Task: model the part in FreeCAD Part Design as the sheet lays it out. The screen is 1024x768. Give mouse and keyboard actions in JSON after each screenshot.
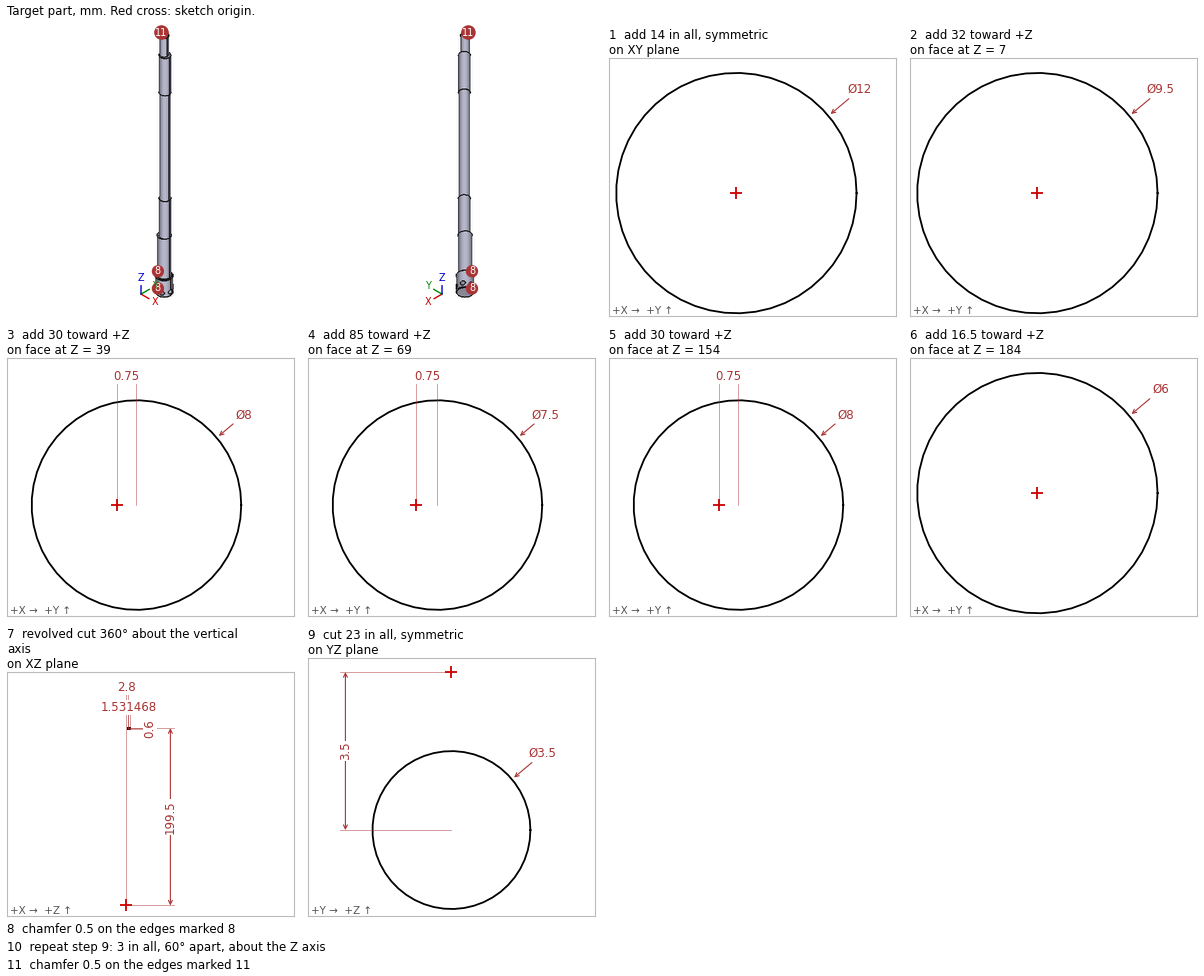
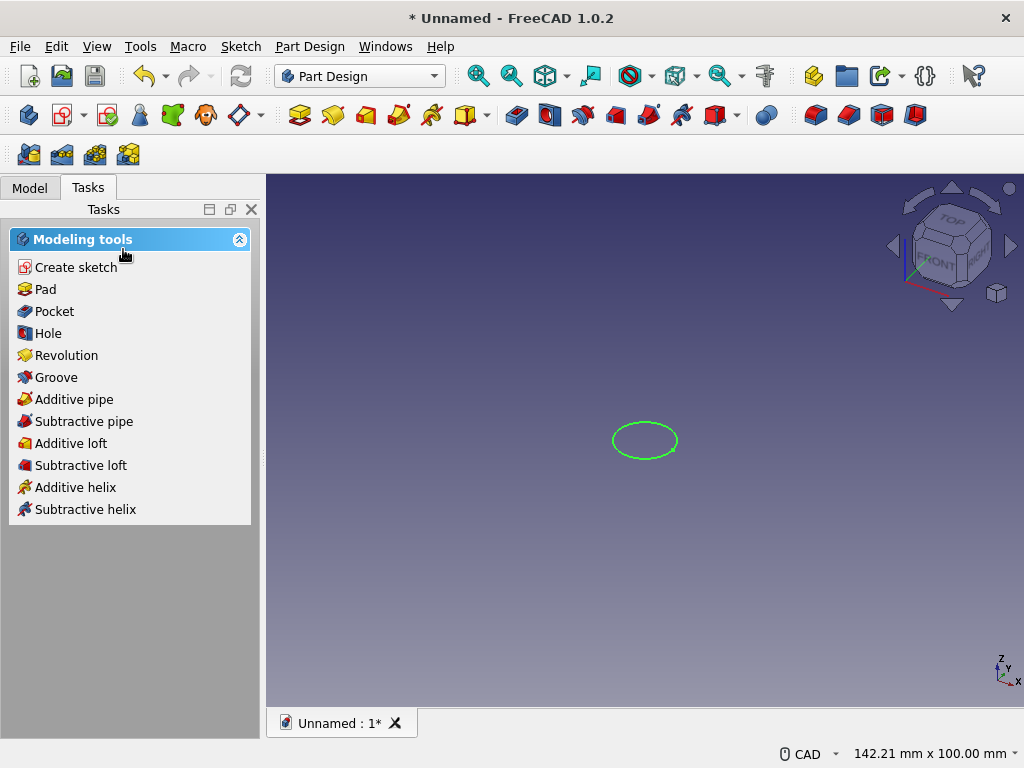
{"action": "left_click", "coordinate": [300, 116]}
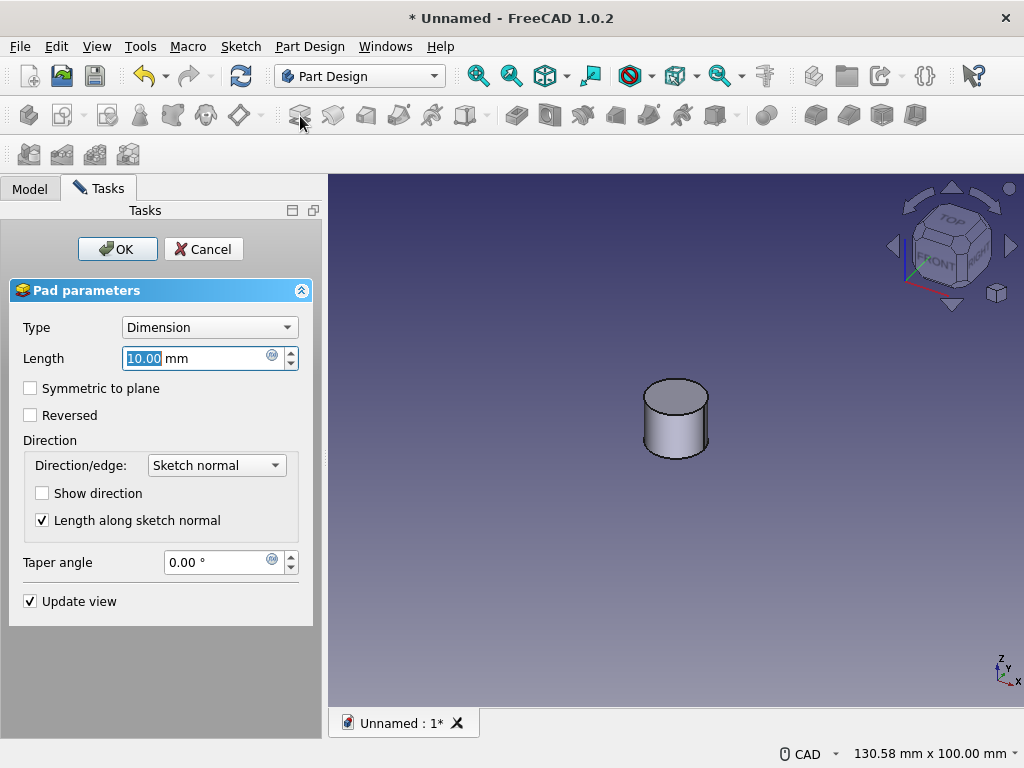
{"action": "type", "text": "14"}
{"action": "key", "text": "Tab"}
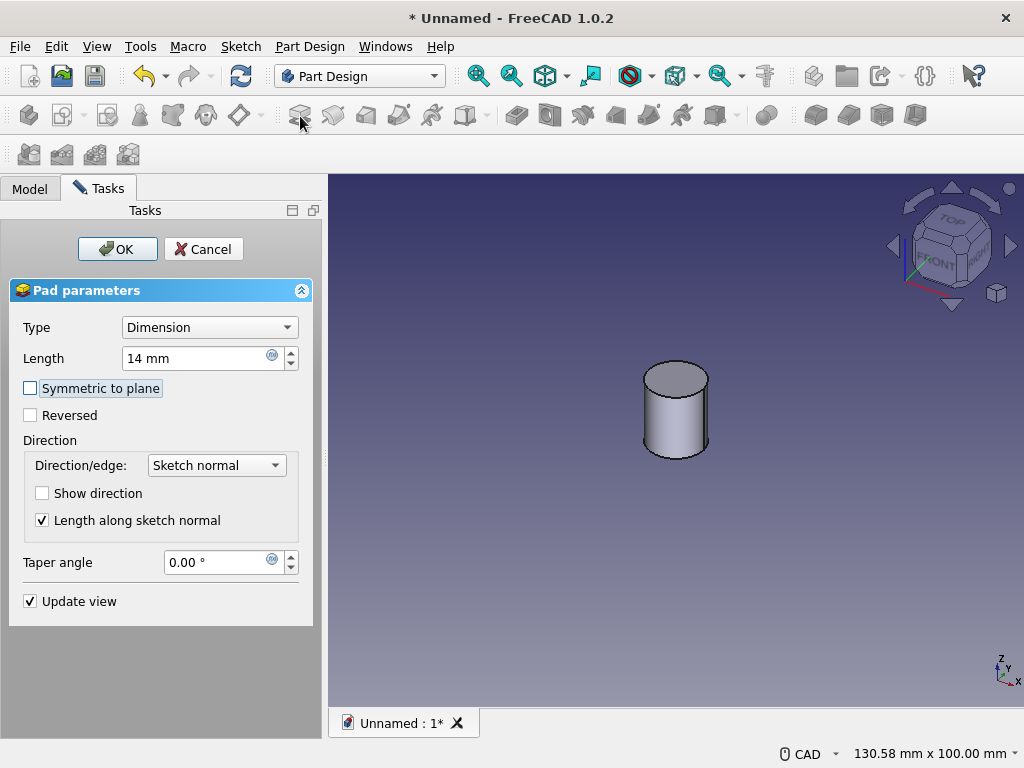
{"action": "left_click", "coordinate": [31, 388]}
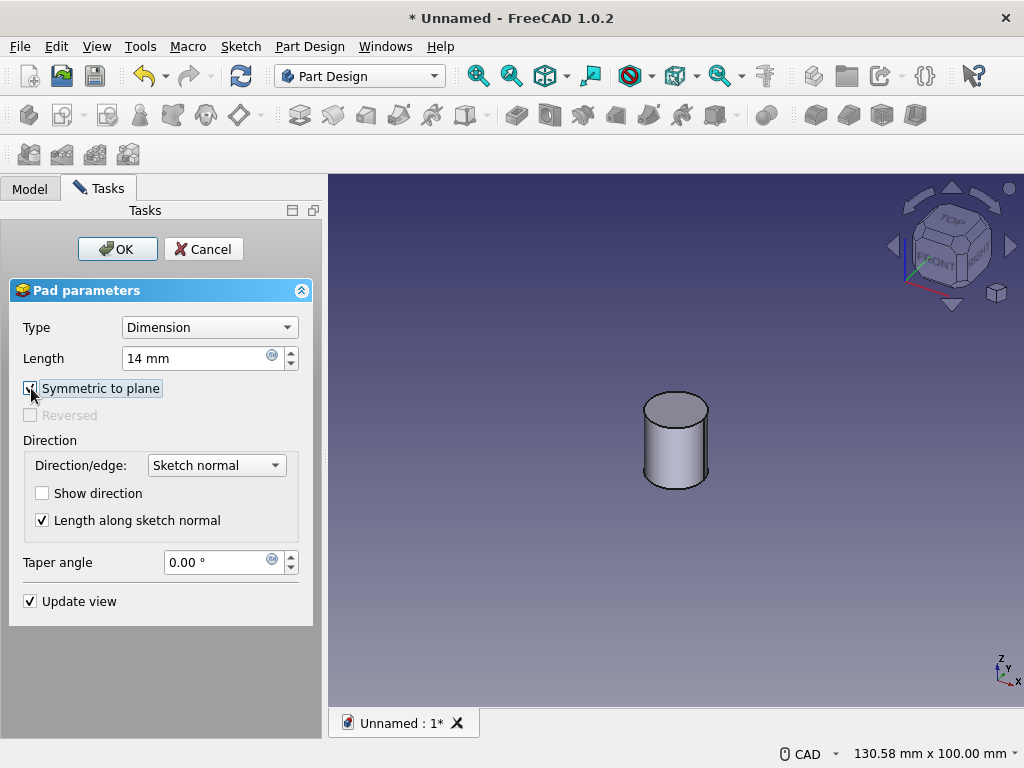
{"action": "left_click", "coordinate": [118, 249]}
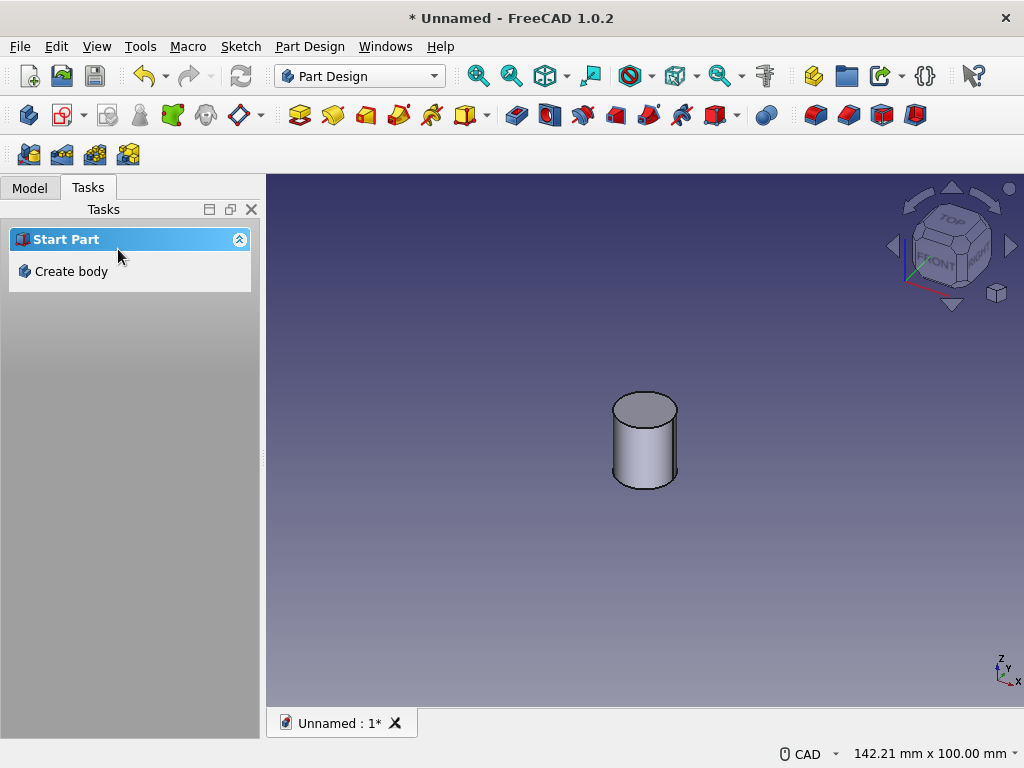
{"action": "left_click", "coordinate": [479, 76]}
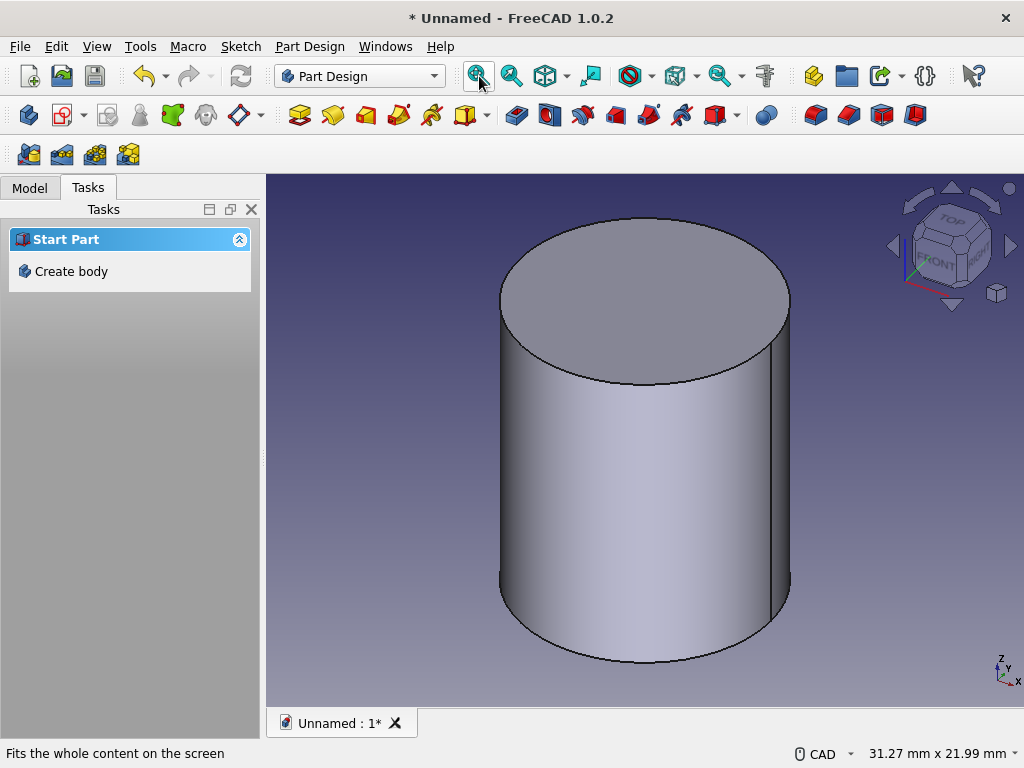
{"action": "left_click", "coordinate": [645, 300]}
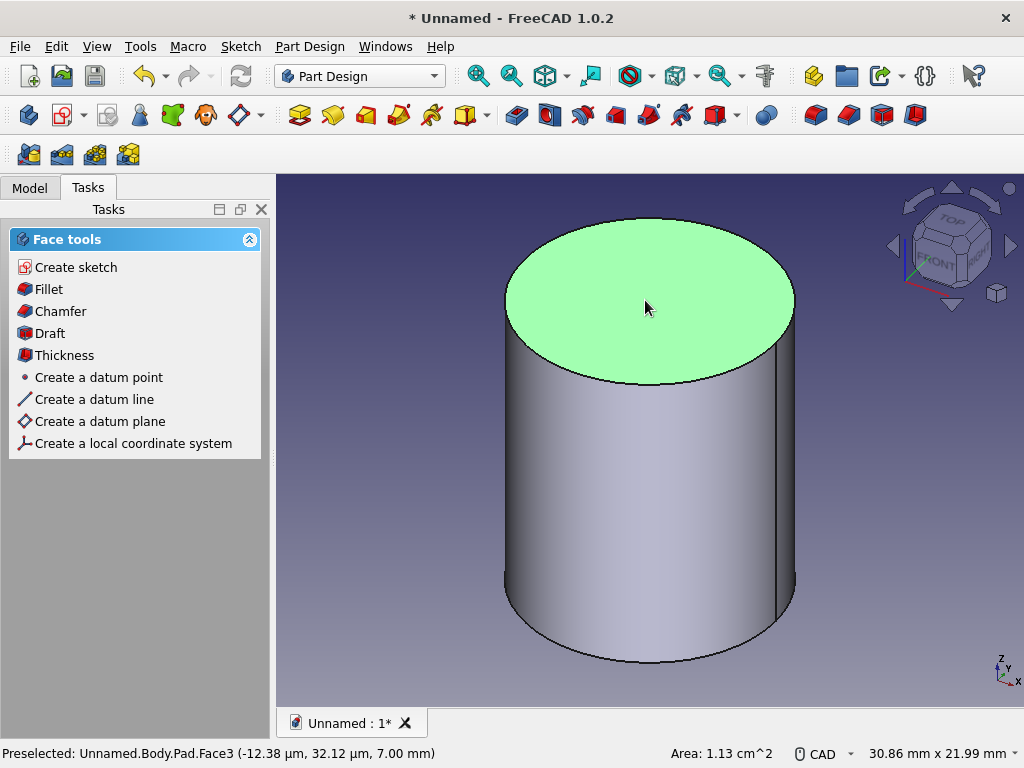
{"action": "left_click", "coordinate": [62, 116]}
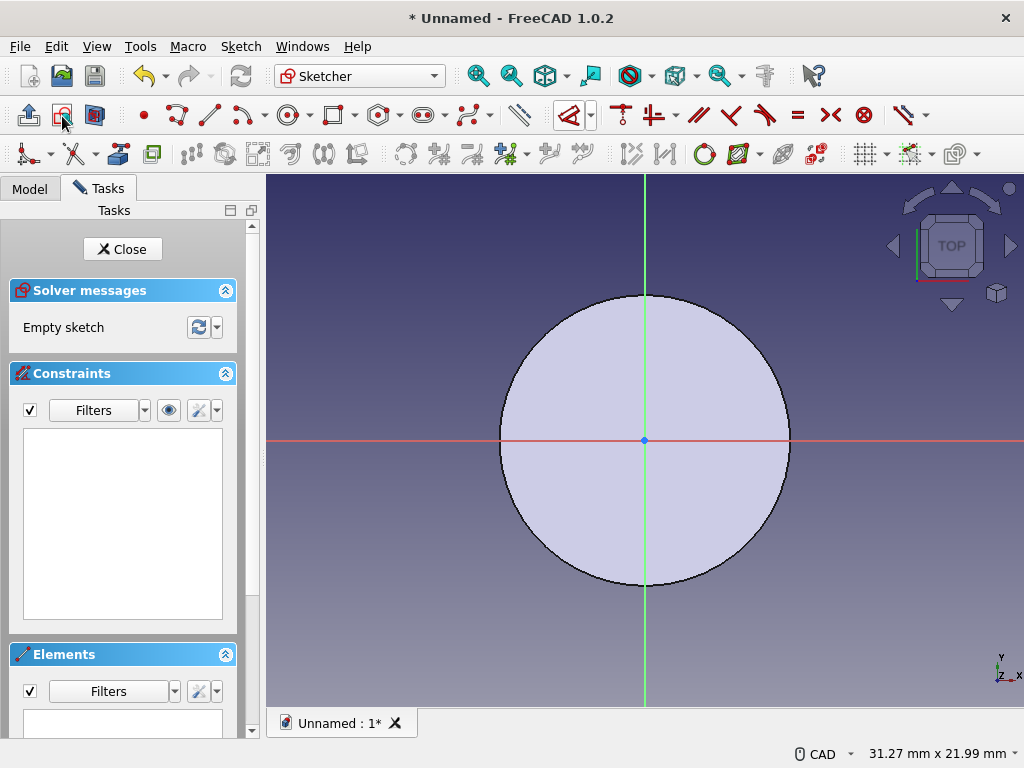
{"action": "scroll", "coordinate": [784, 440], "scroll_direction": "up", "scroll_amount": 2}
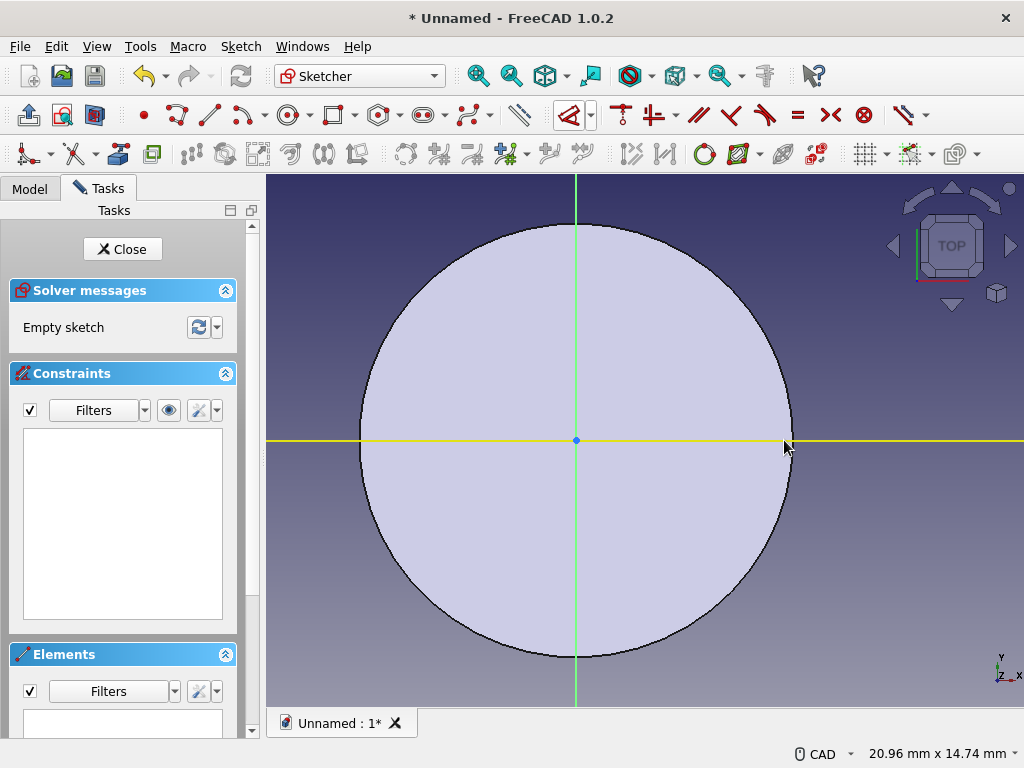
{"action": "key", "text": "g c"}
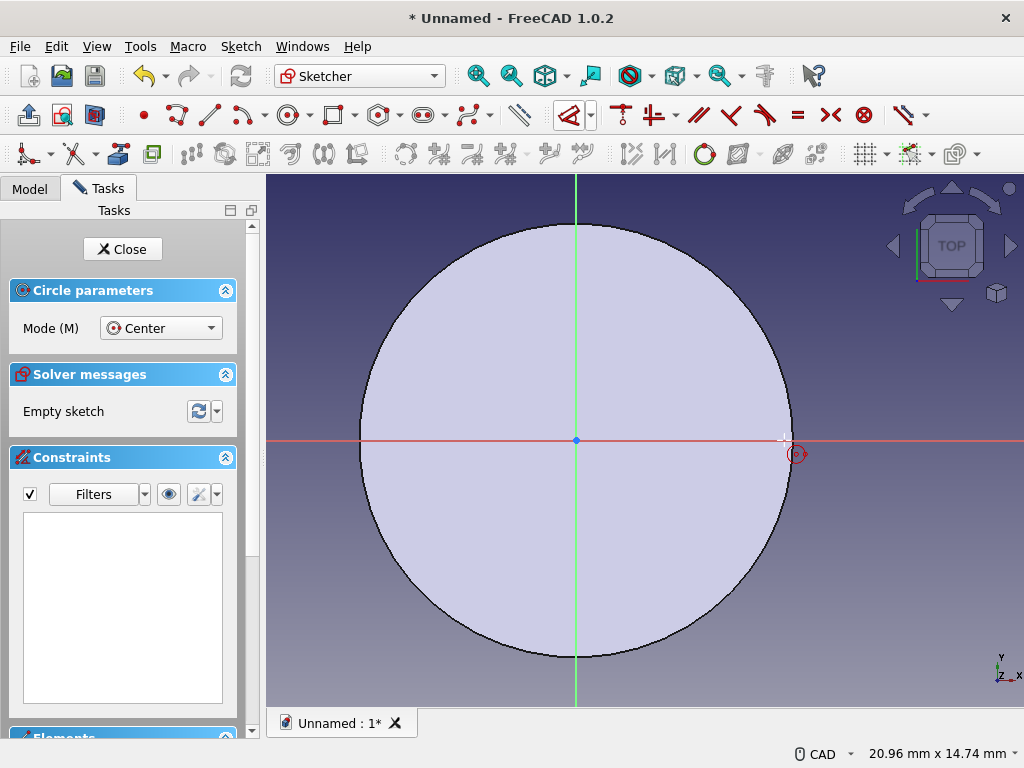
{"action": "left_click", "coordinate": [576, 440]}
{"action": "left_click", "coordinate": [698, 319]}
{"action": "key", "text": "Escape"}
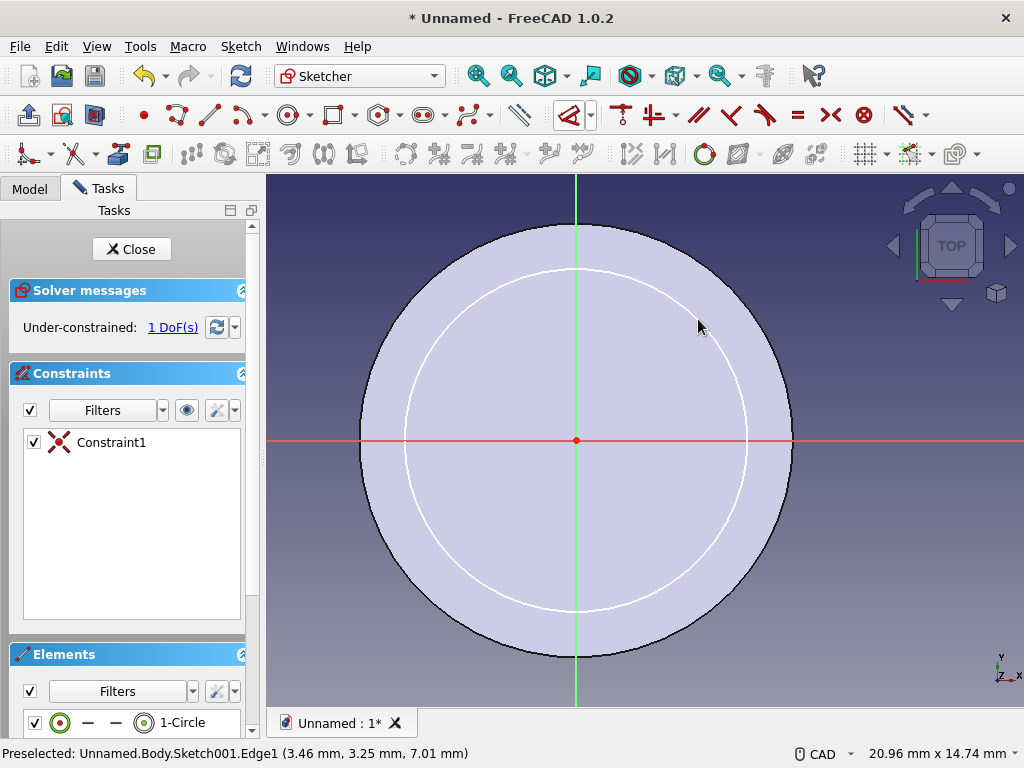
{"action": "left_click", "coordinate": [697, 319]}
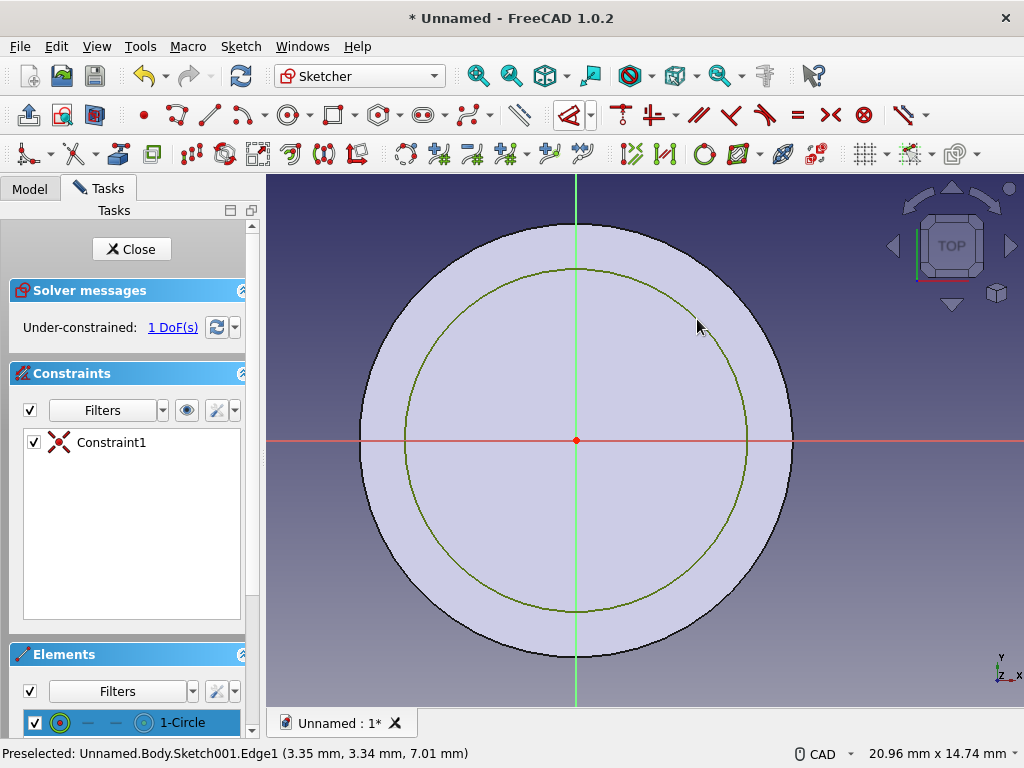
{"action": "key", "text": "k o"}